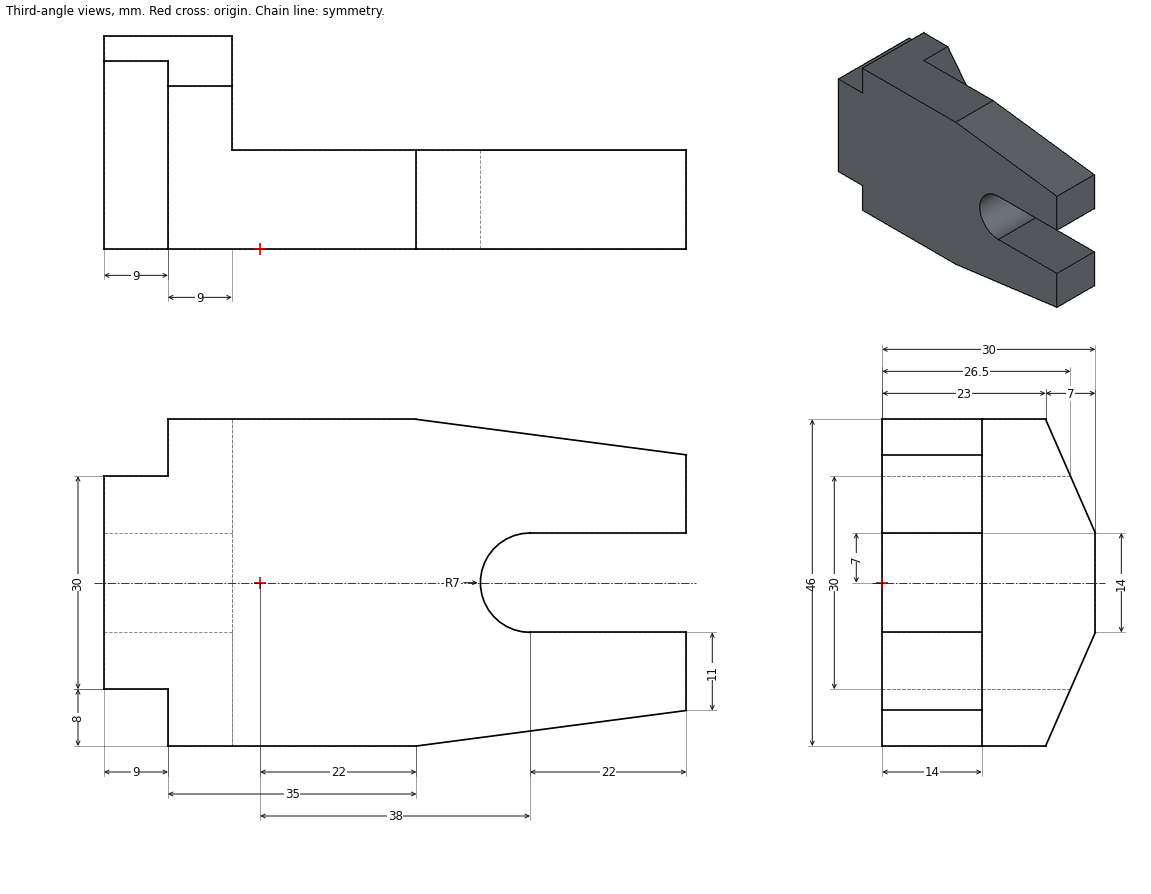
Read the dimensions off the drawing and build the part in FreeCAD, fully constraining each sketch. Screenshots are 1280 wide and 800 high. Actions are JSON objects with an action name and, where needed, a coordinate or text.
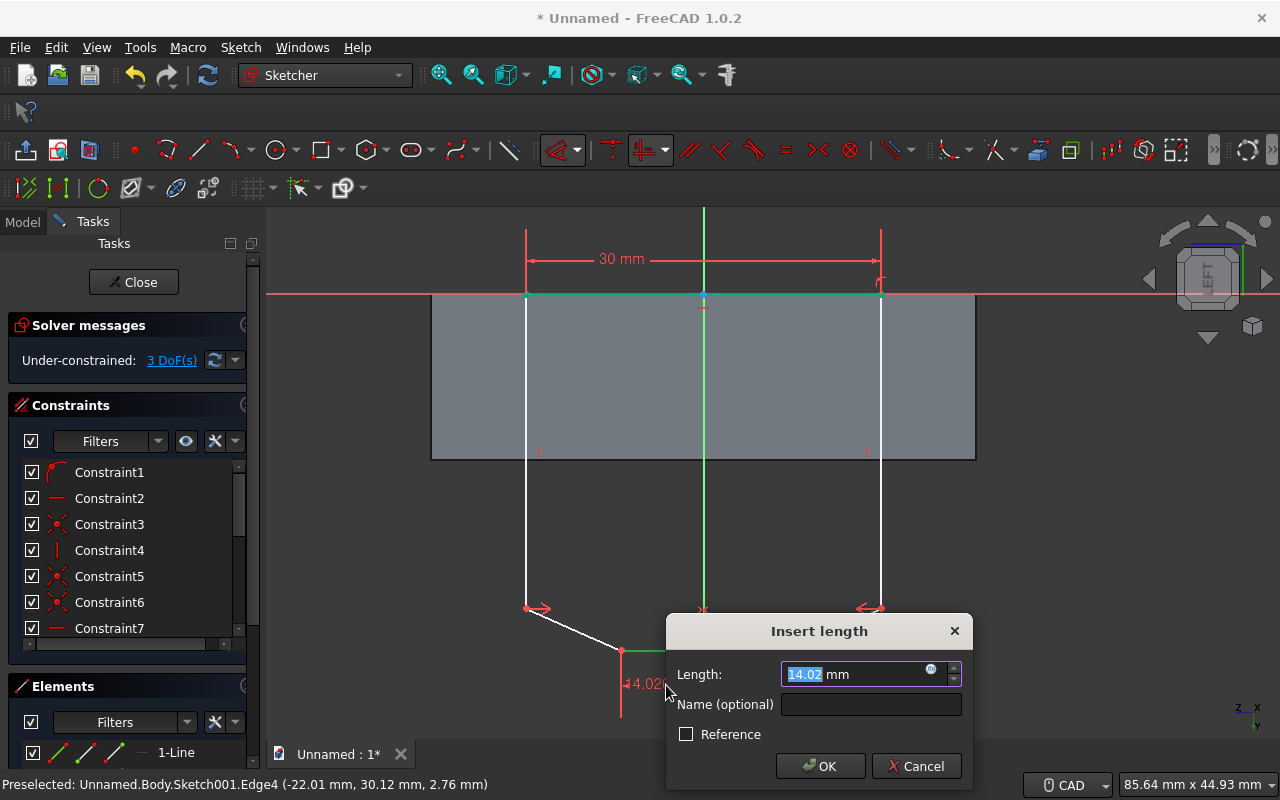
{"action": "type", "text": "14"}
{"action": "key", "text": "Return"}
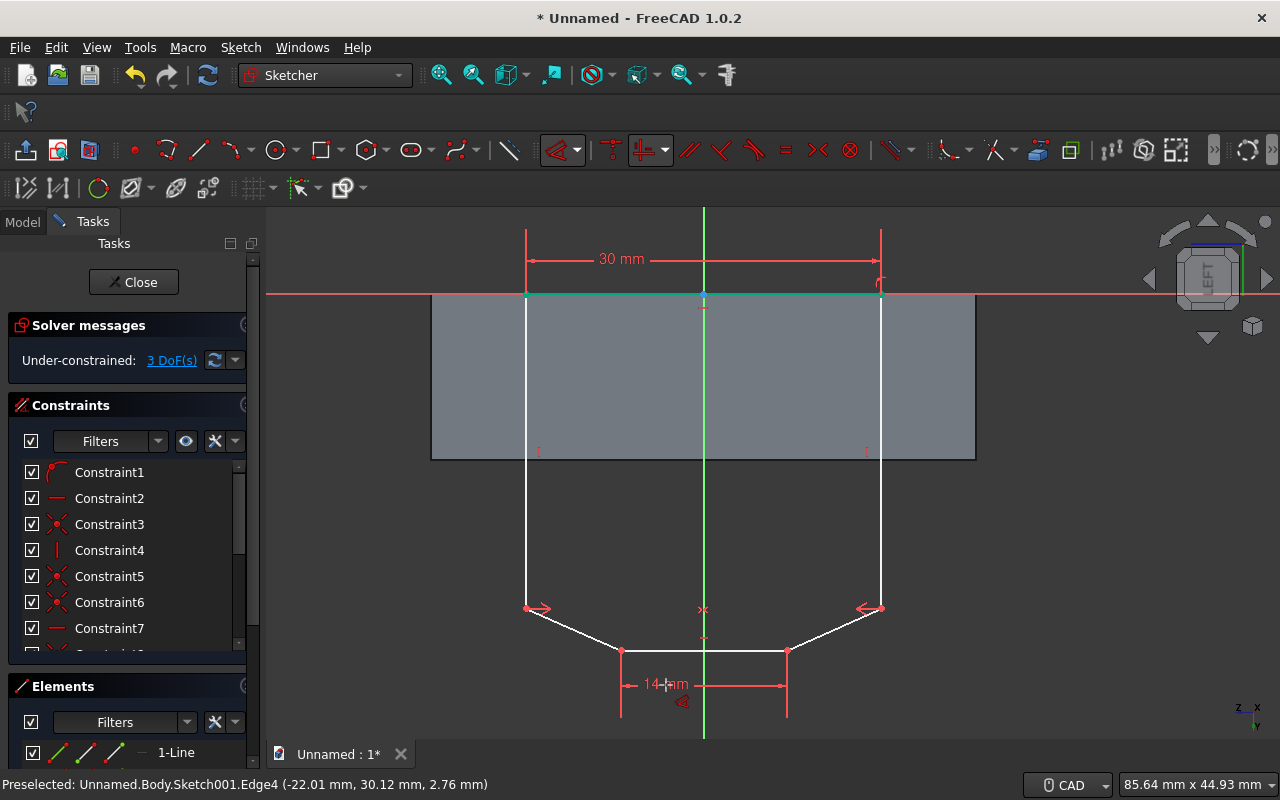
{"action": "left_click", "coordinate": [621, 651]}
{"action": "left_click", "coordinate": [662, 709]}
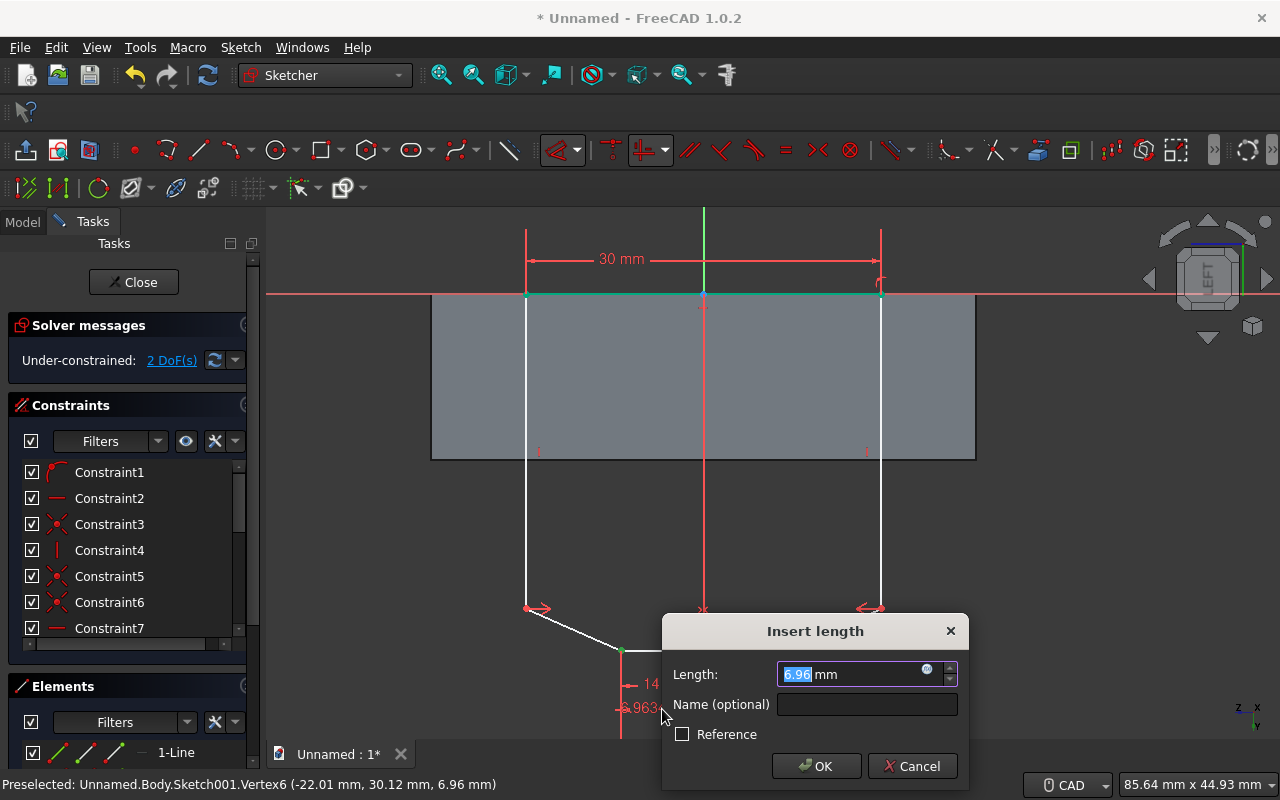
{"action": "type", "text": "7"}
{"action": "key", "text": "Return"}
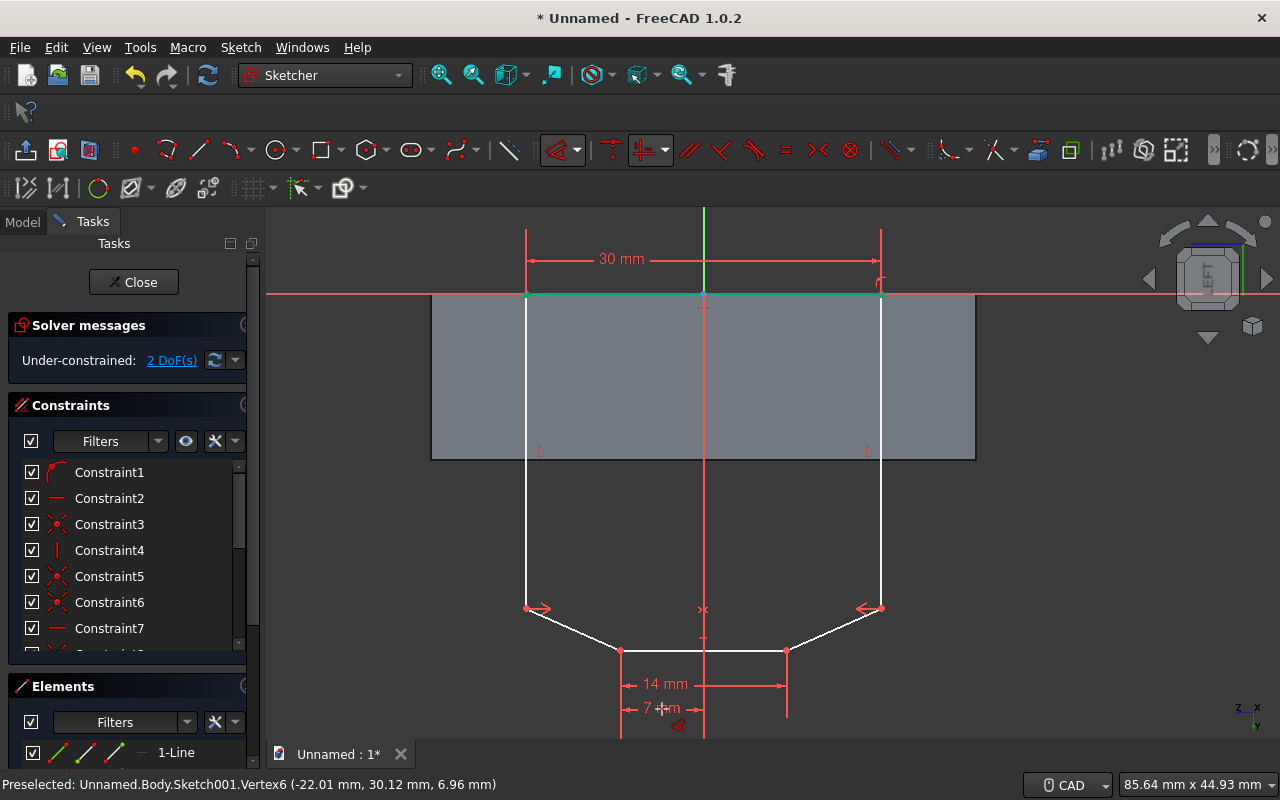
{"action": "left_click", "coordinate": [621, 651]}
{"action": "left_click", "coordinate": [587, 473]}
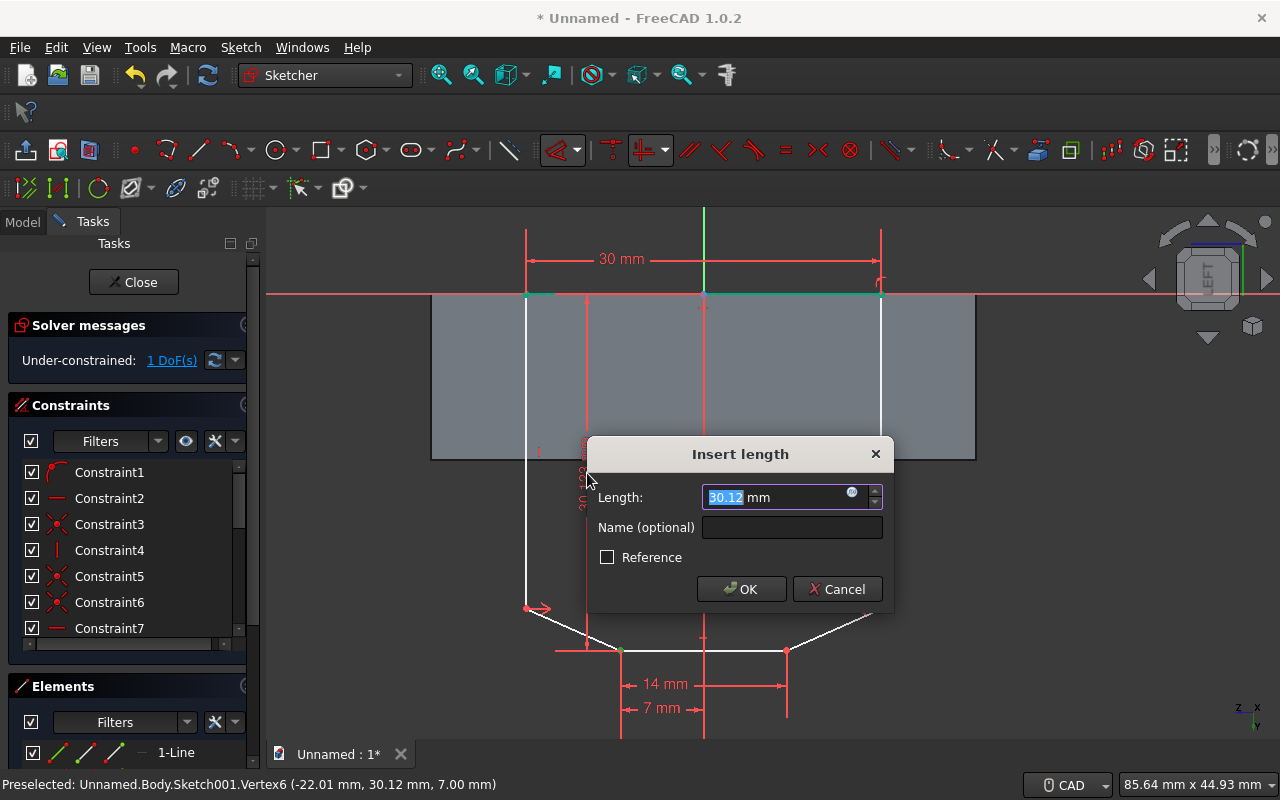
{"action": "type", "text": "30"}
{"action": "key", "text": "Return"}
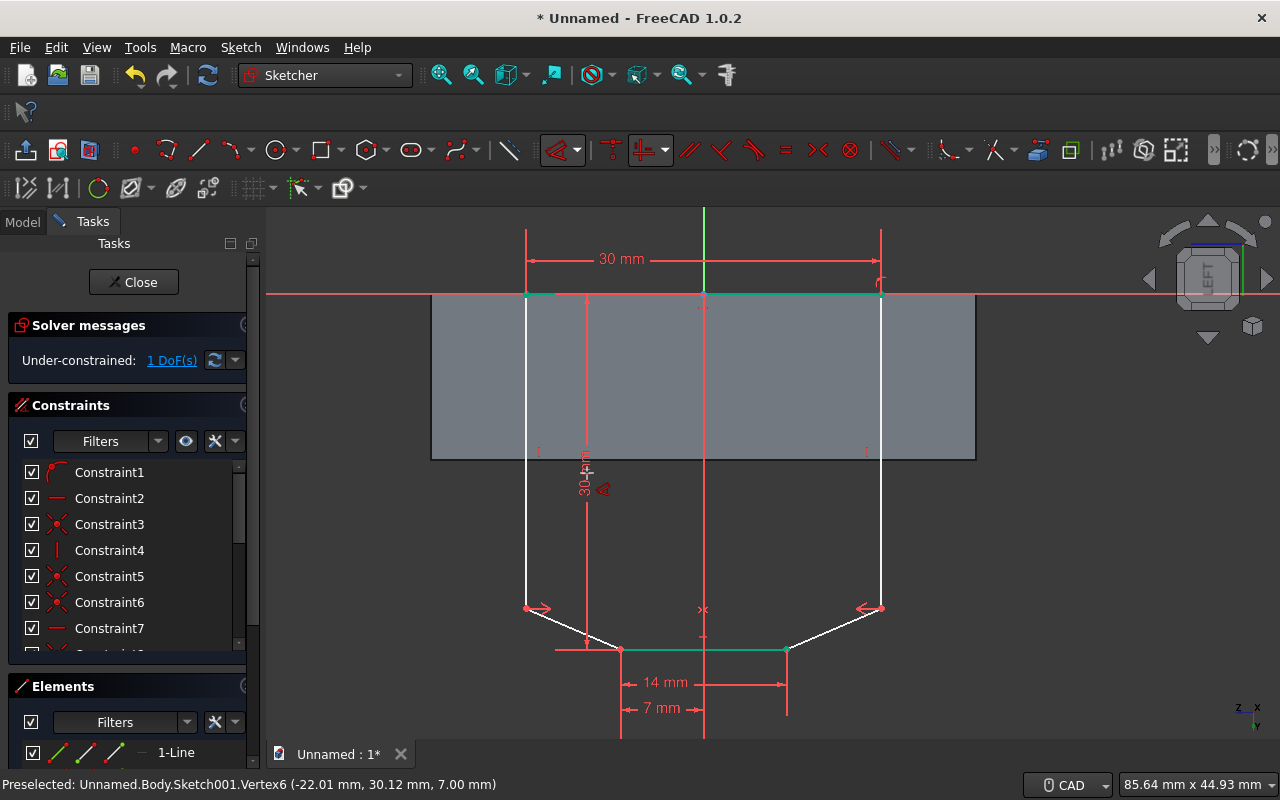
{"action": "left_click", "coordinate": [526, 389]}
{"action": "left_click", "coordinate": [492, 452]}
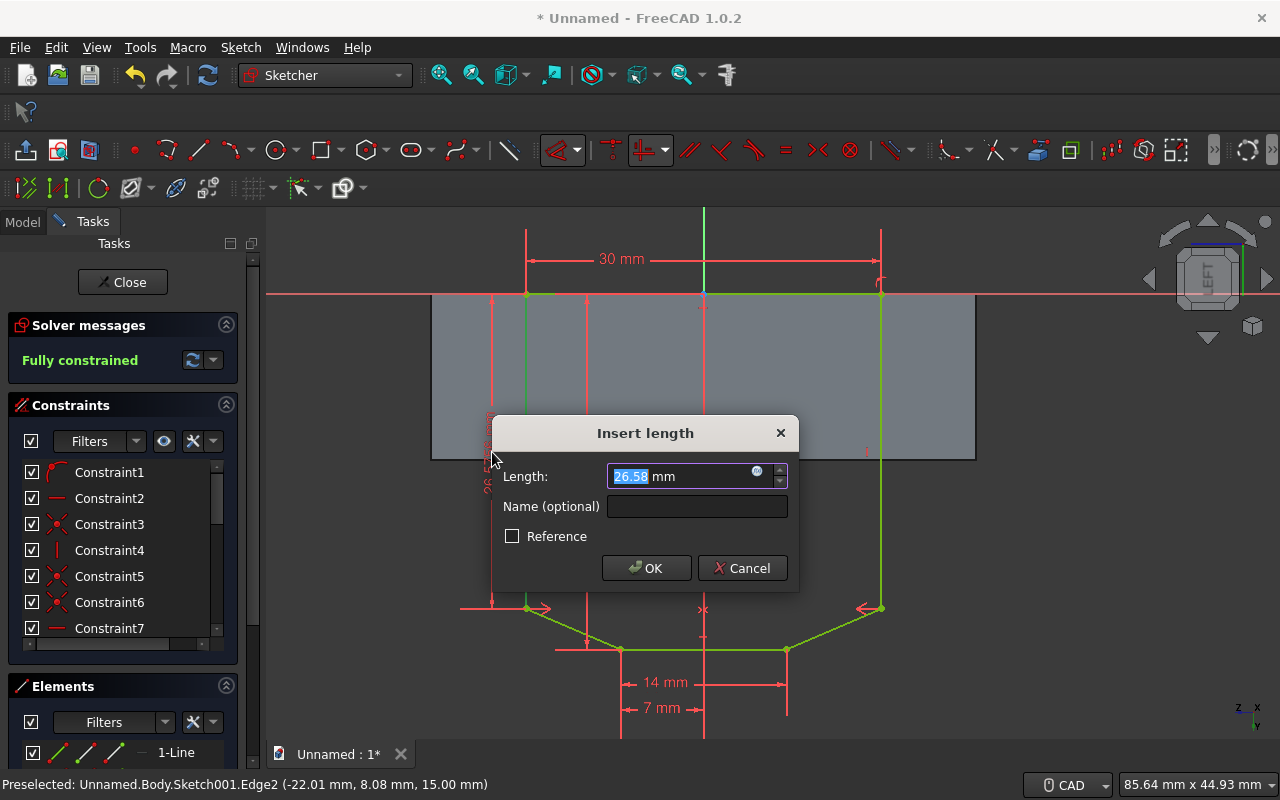
{"action": "type", "text": "26.5"}
{"action": "key", "text": "Return"}
{"action": "key", "text": "Escape"}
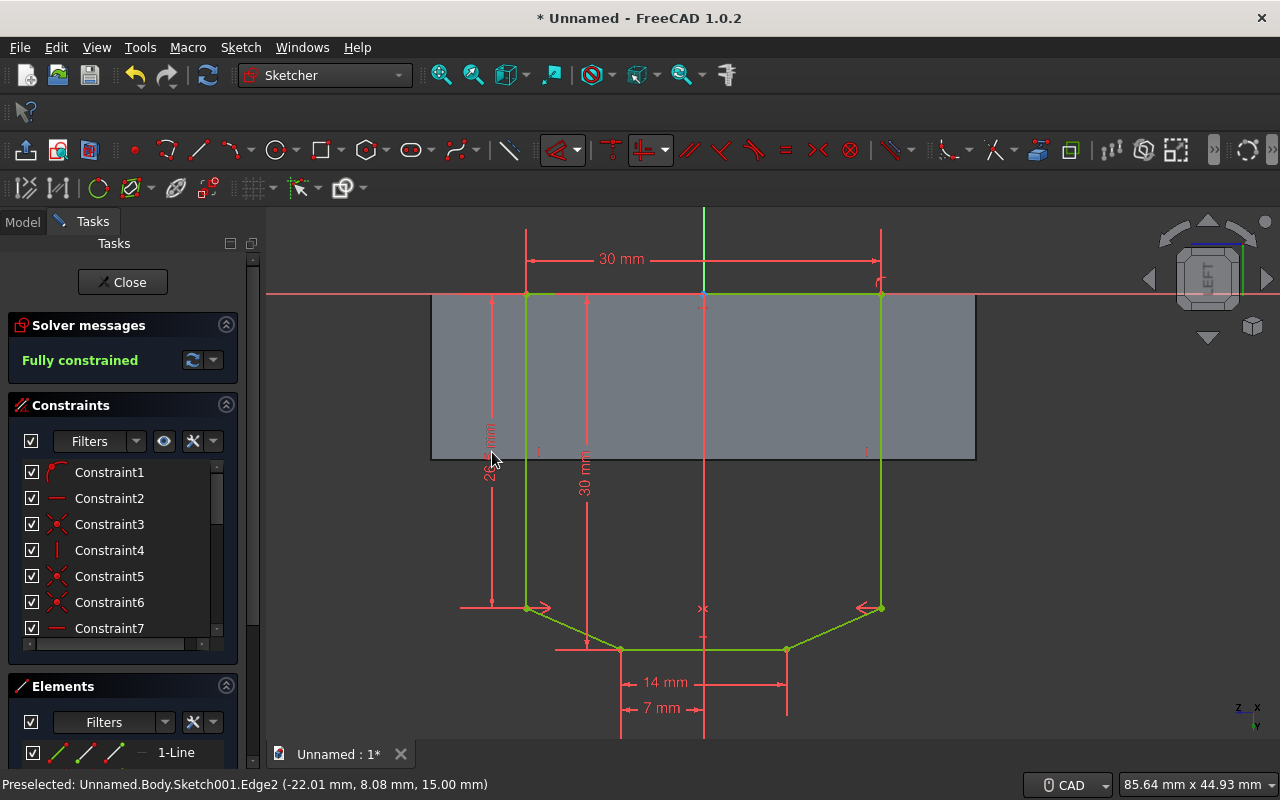
{"action": "left_click", "coordinate": [123, 282]}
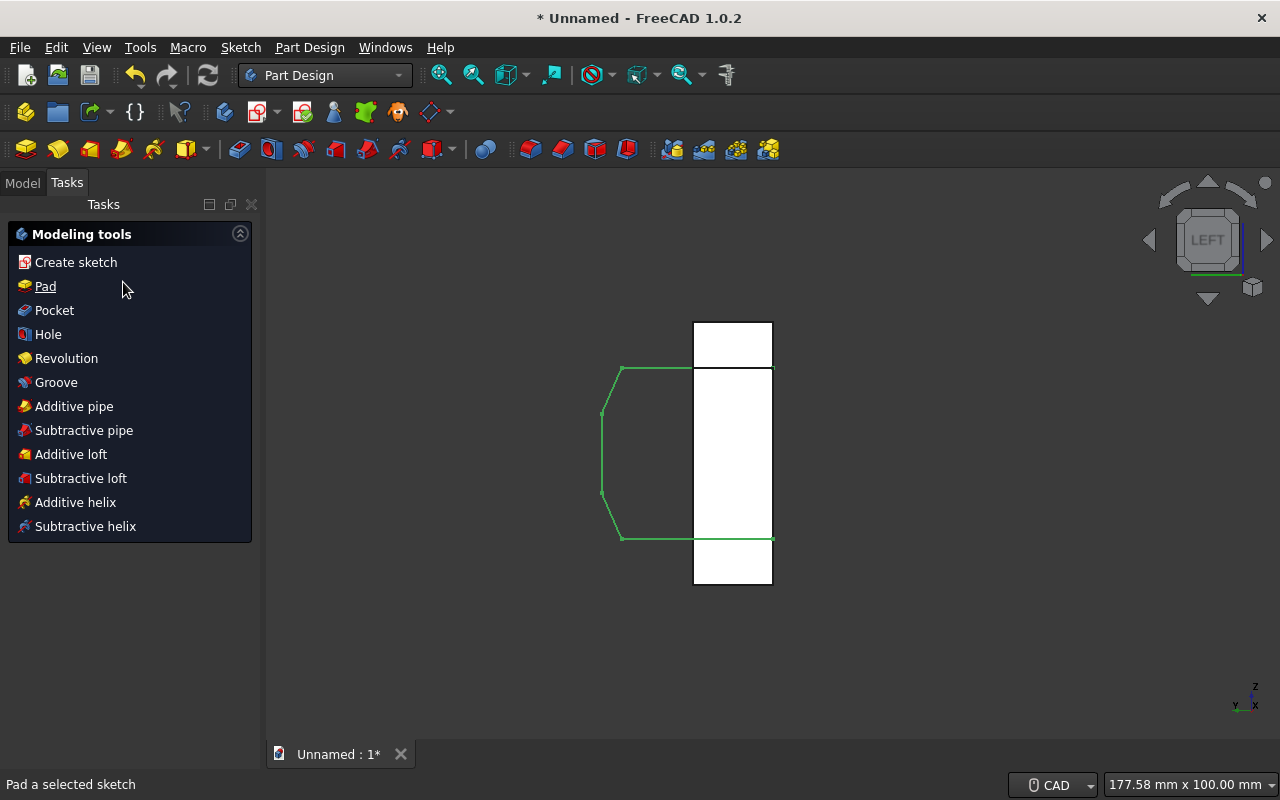
{"action": "left_click", "coordinate": [26, 150]}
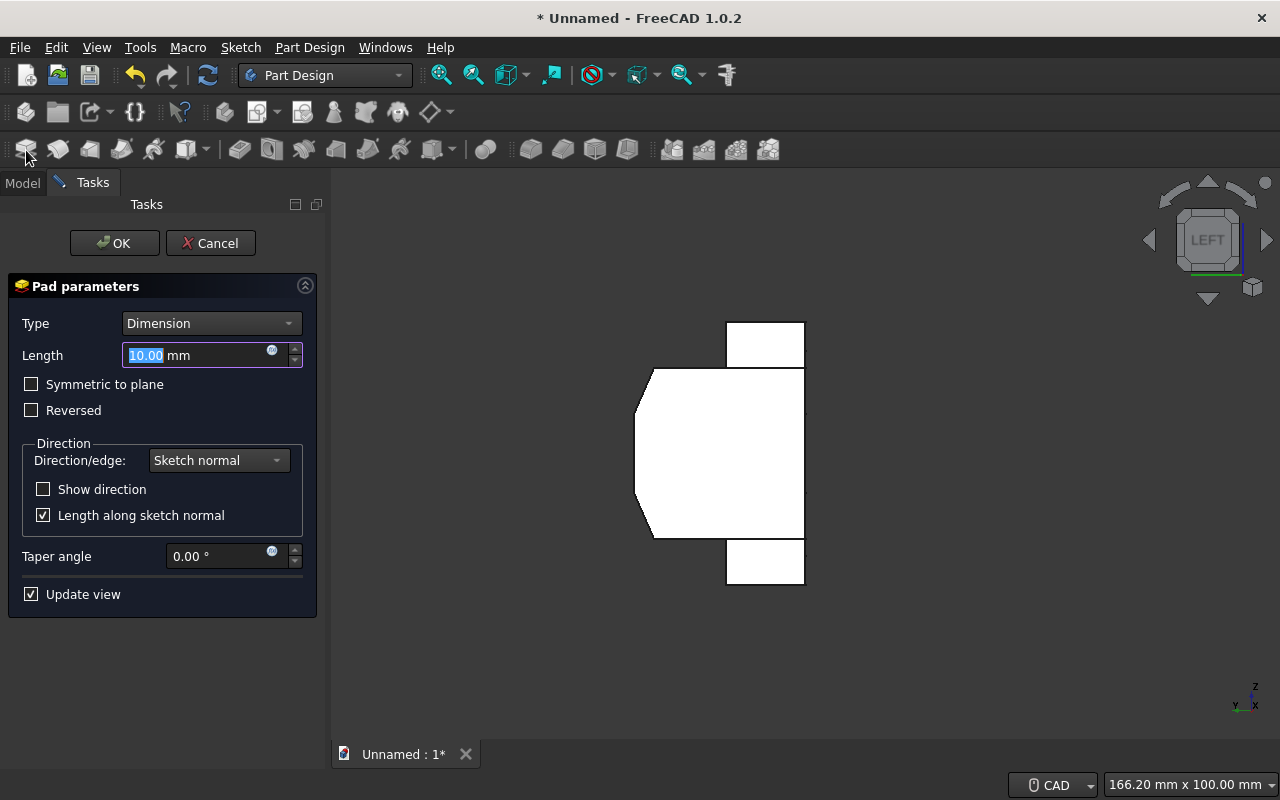
{"action": "type", "text": "9"}
{"action": "key", "text": "Tab"}